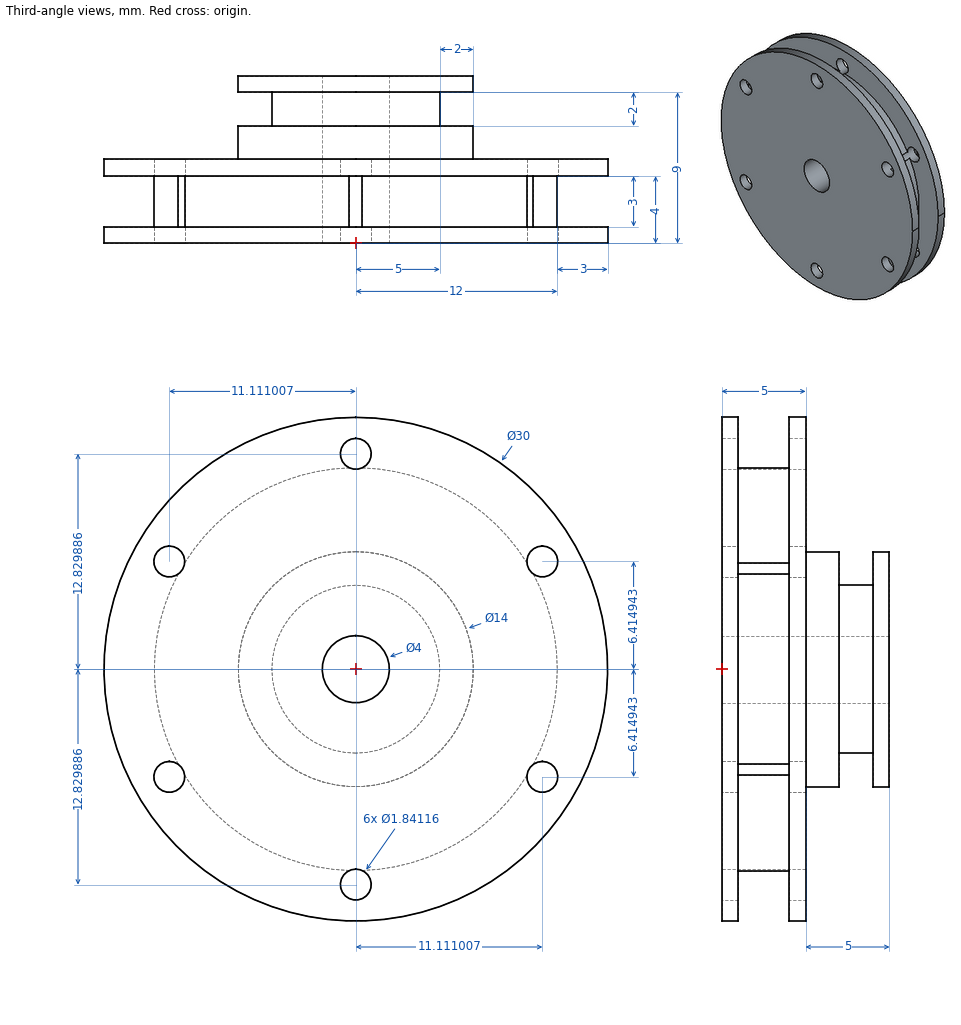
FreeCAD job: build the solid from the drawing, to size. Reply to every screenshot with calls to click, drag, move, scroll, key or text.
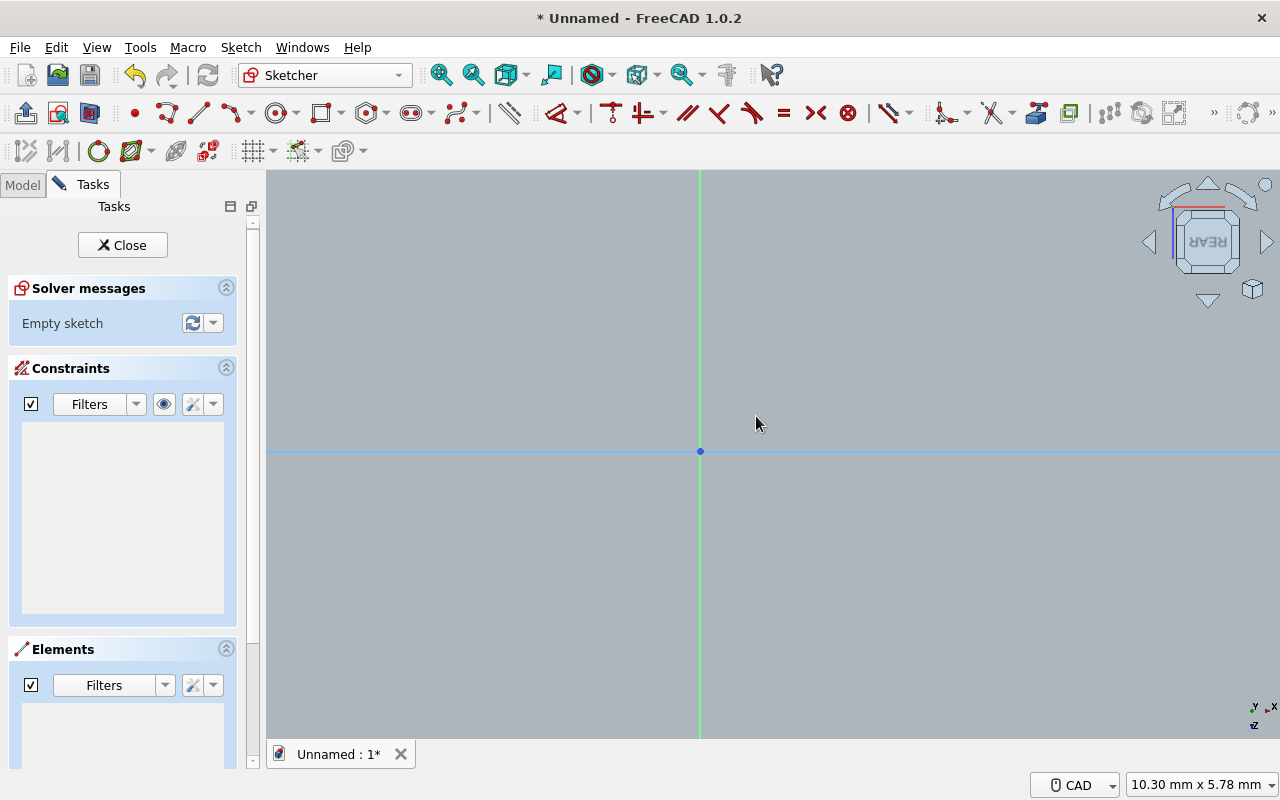
click(276, 114)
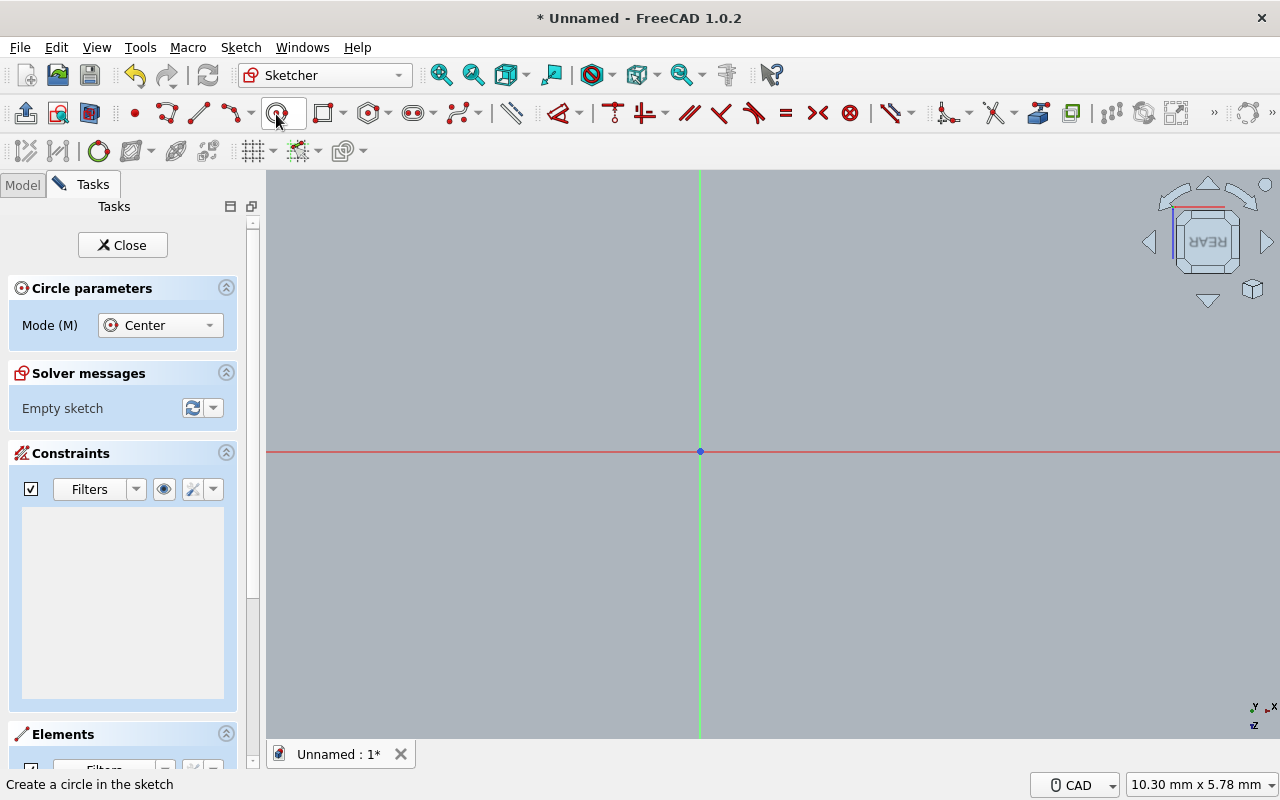
click(700, 452)
move(840, 313)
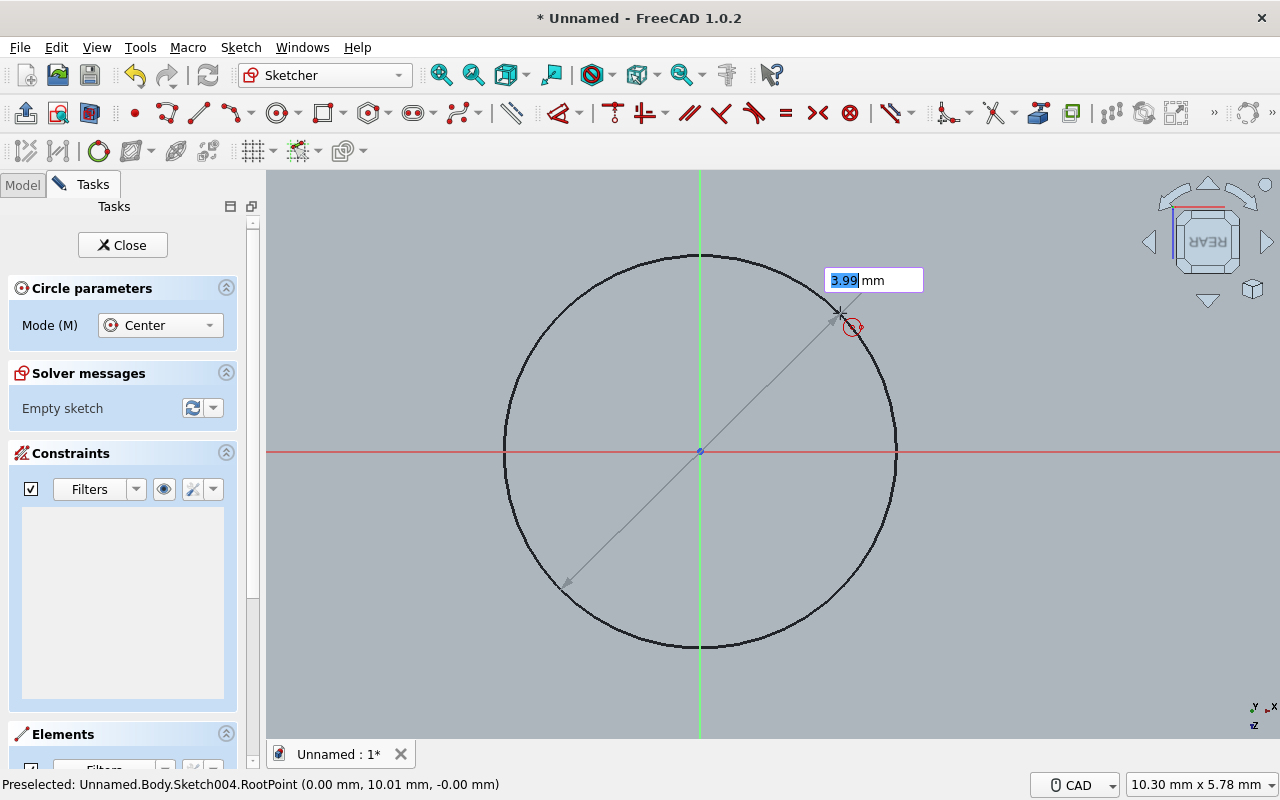
text(4)
key(Return)
key(Escape)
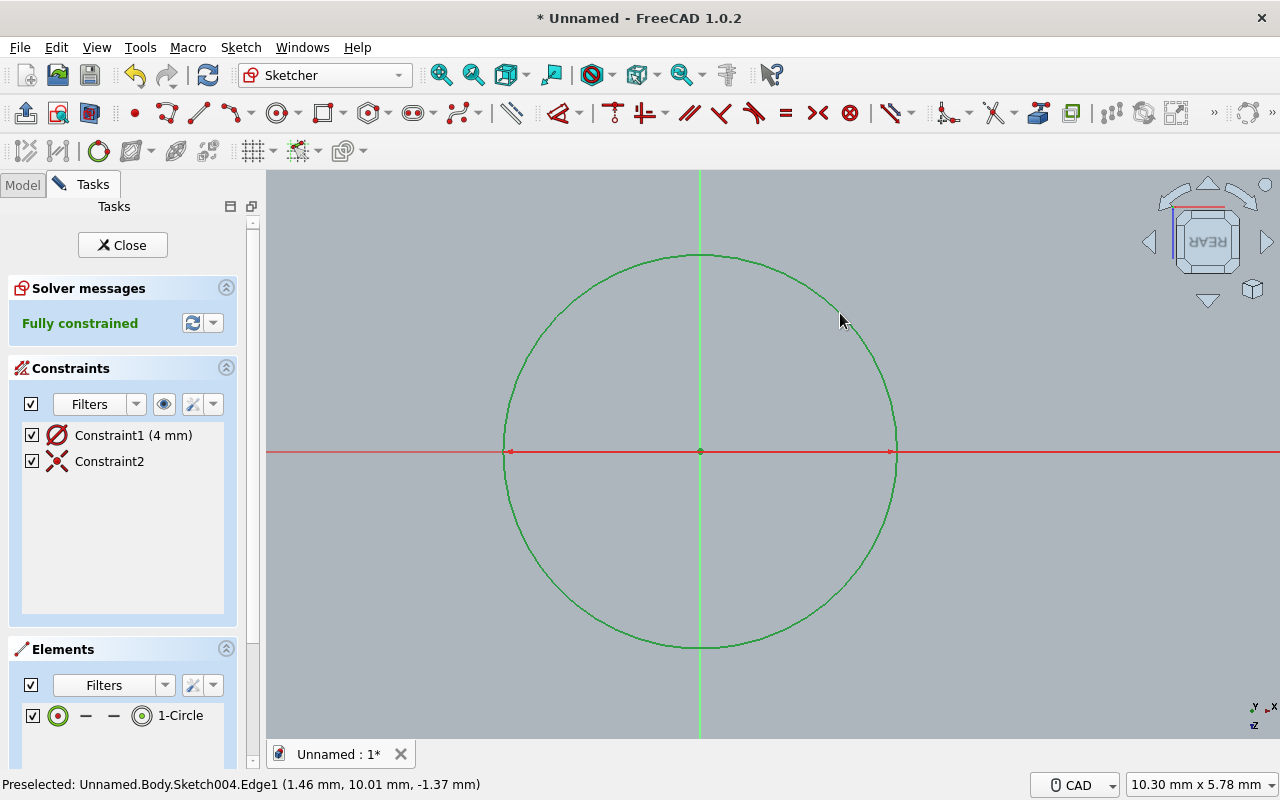
click(123, 245)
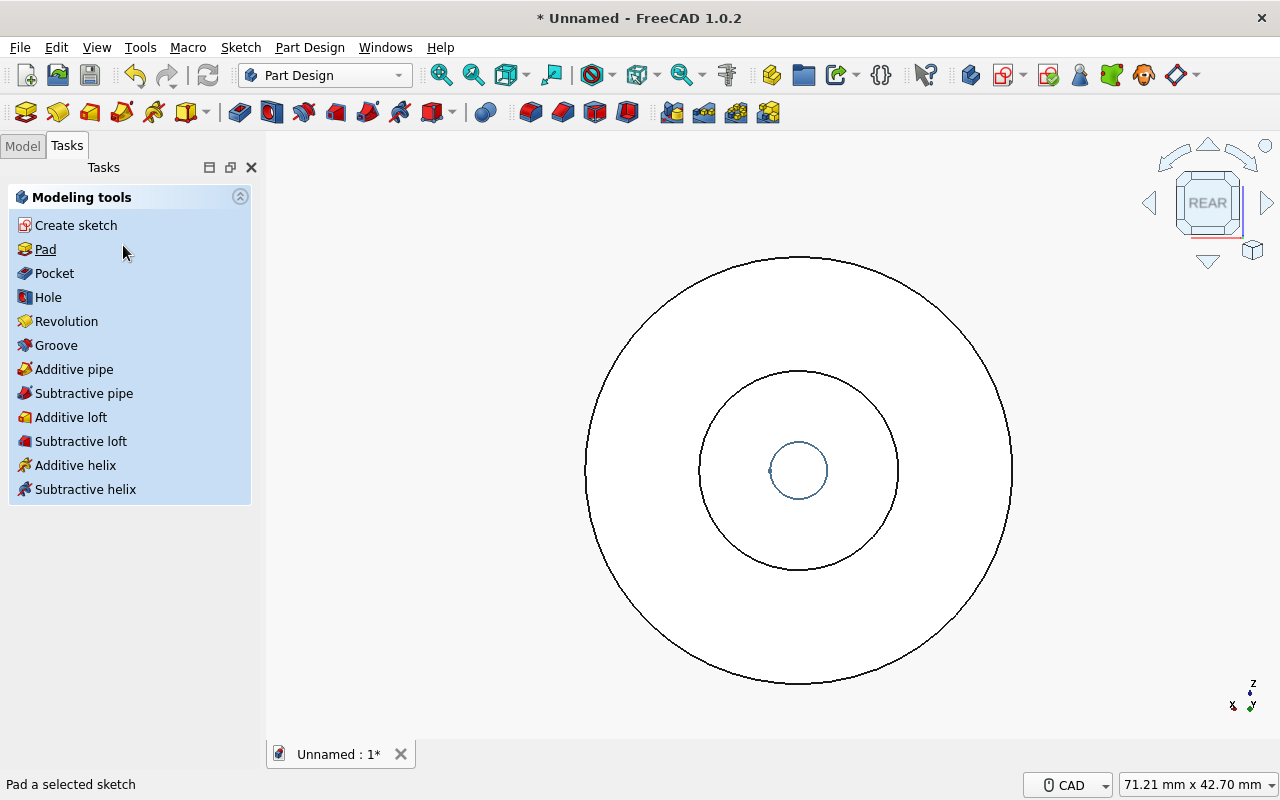
click(240, 112)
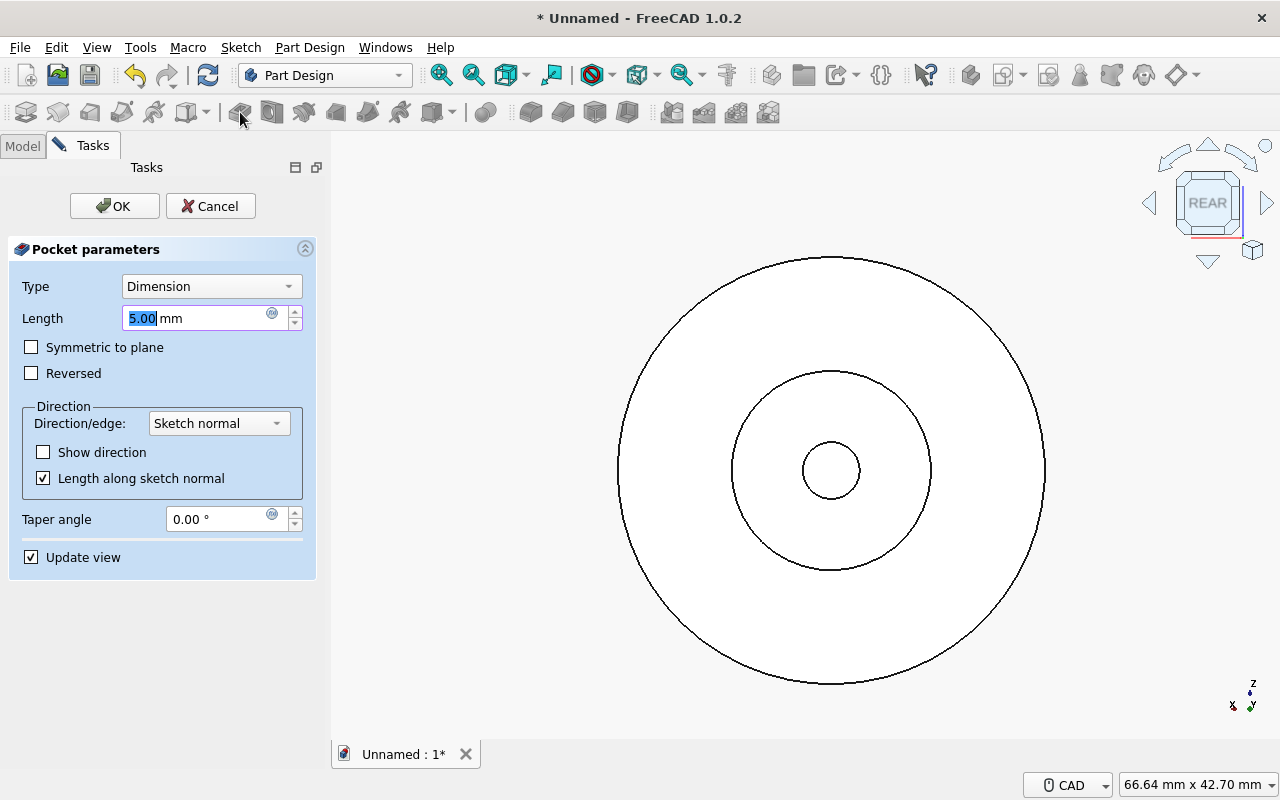
click(212, 286)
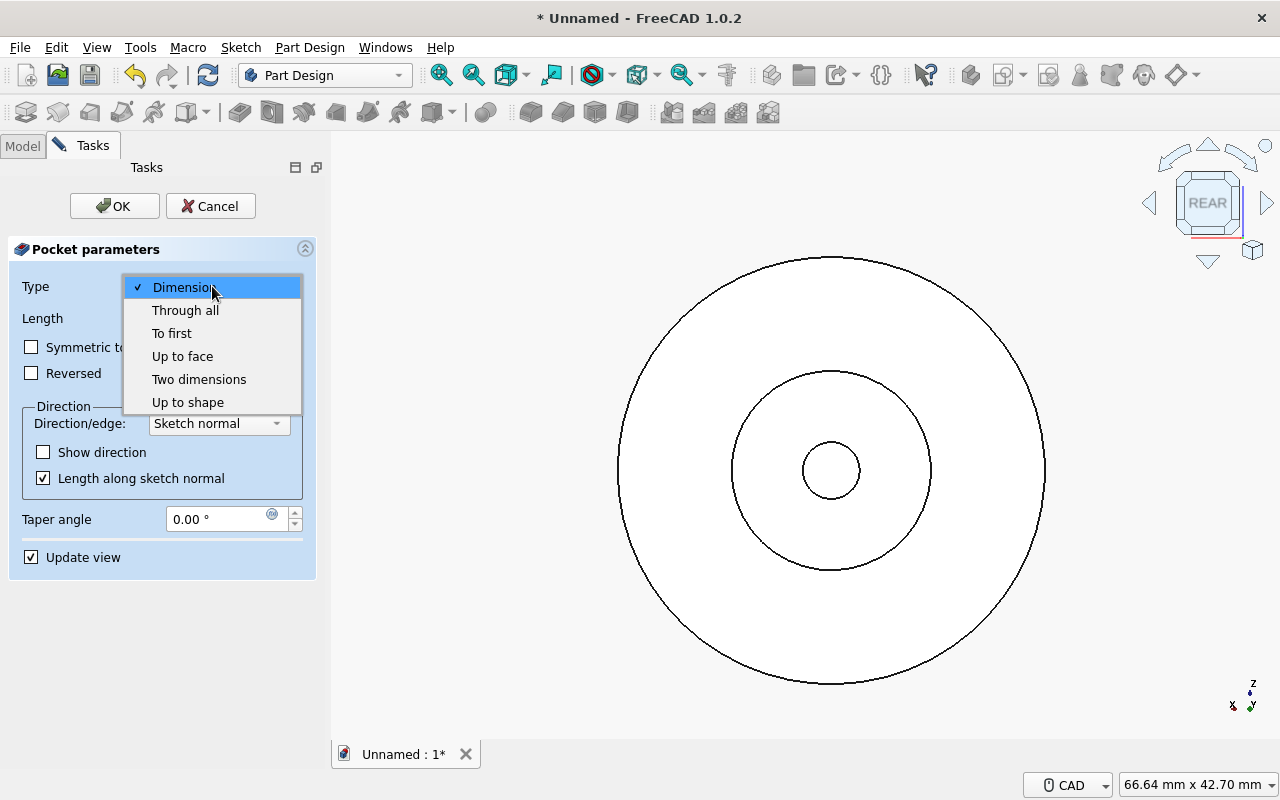
click(212, 310)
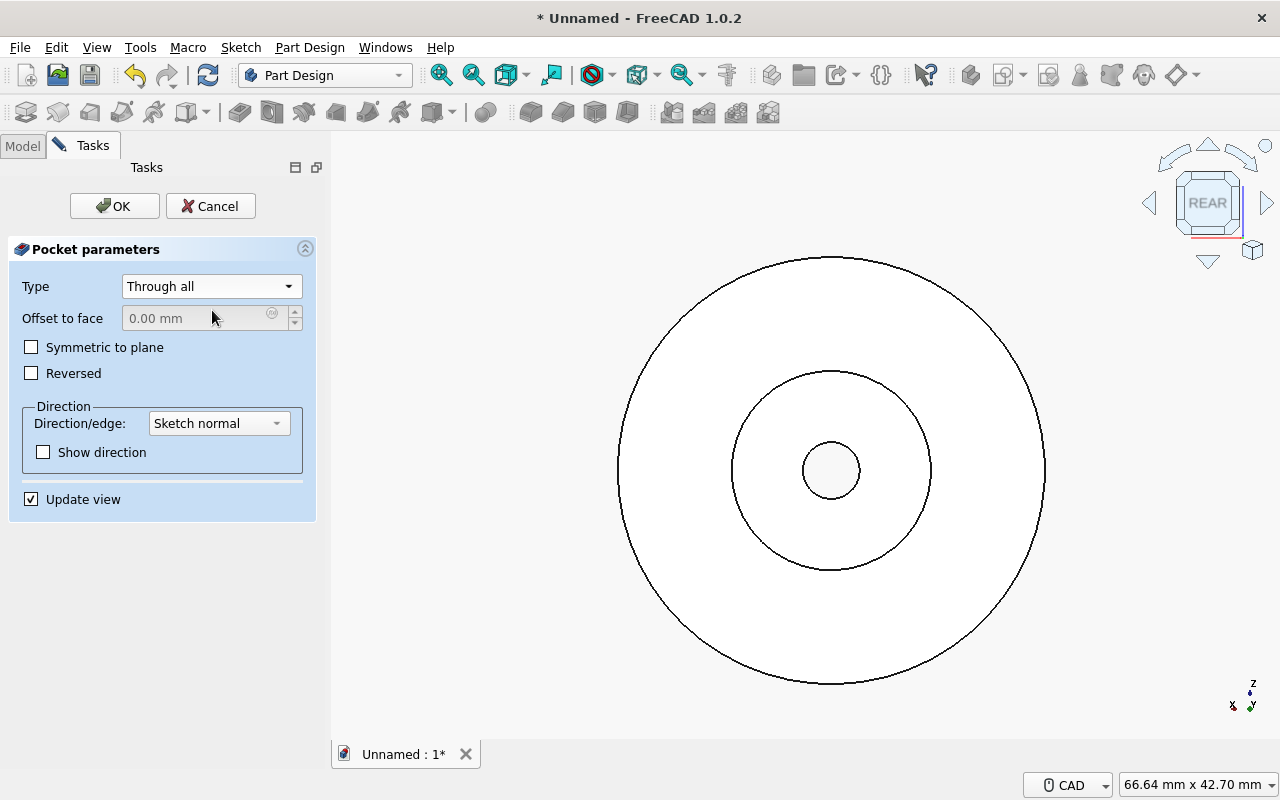
click(115, 206)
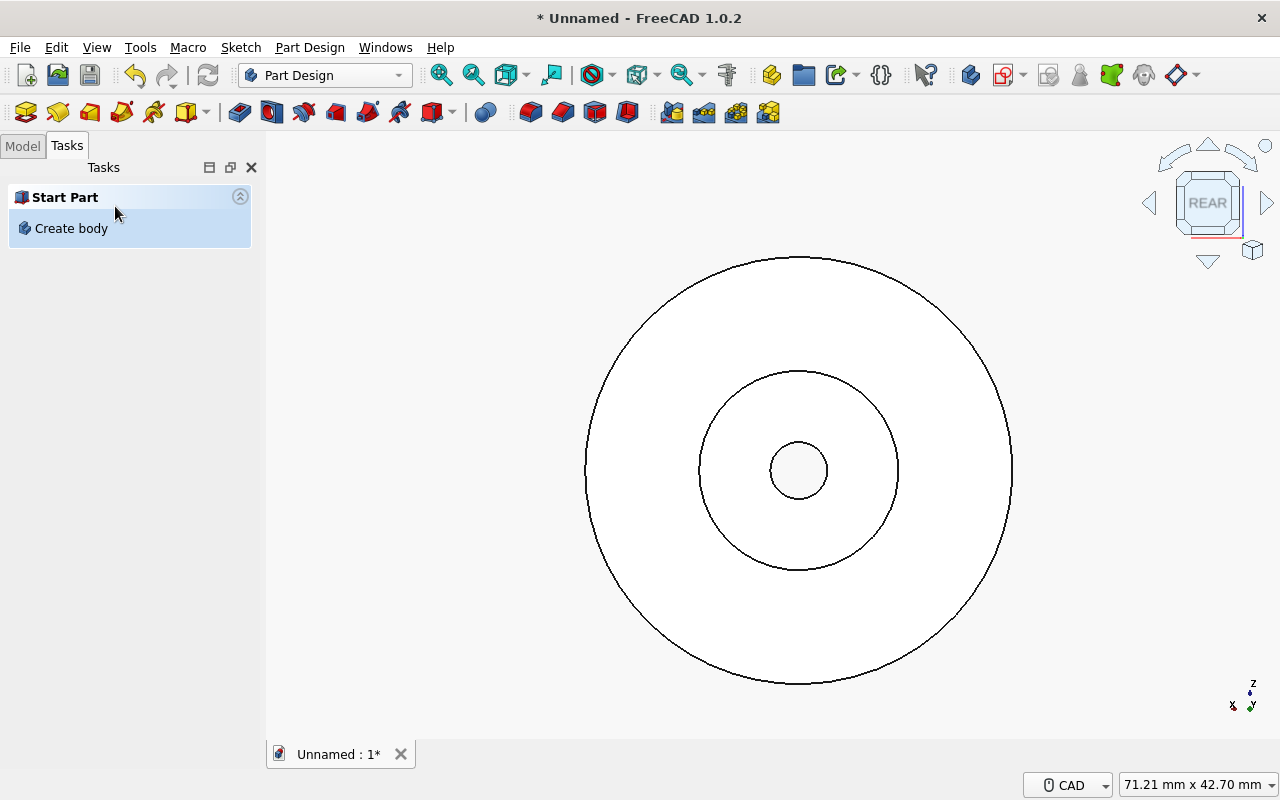
click(921, 592)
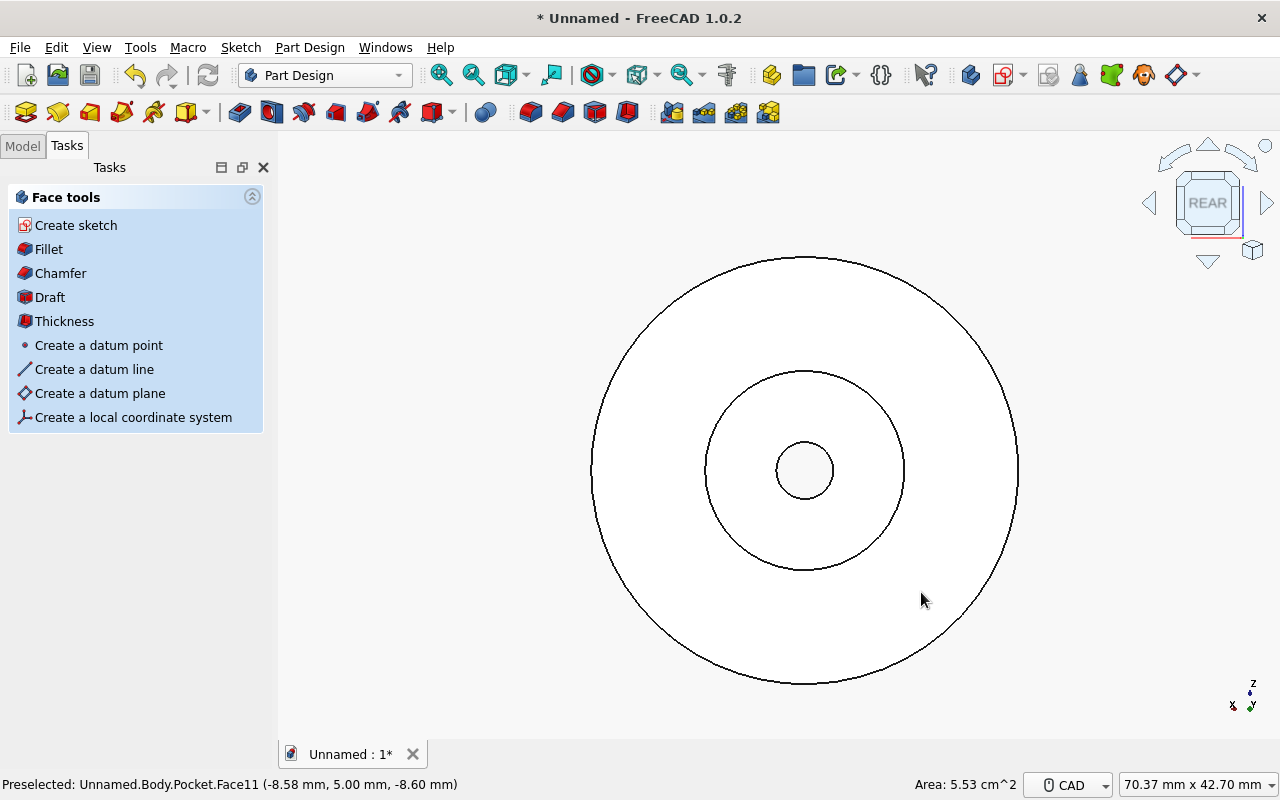
click(1004, 76)